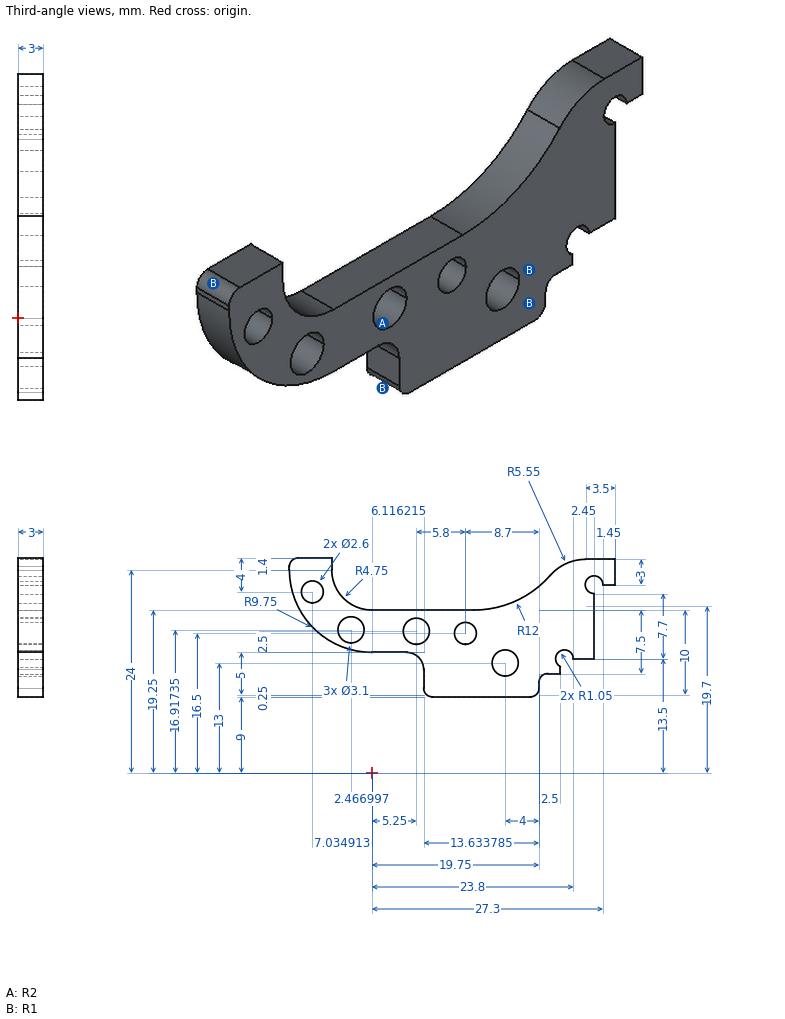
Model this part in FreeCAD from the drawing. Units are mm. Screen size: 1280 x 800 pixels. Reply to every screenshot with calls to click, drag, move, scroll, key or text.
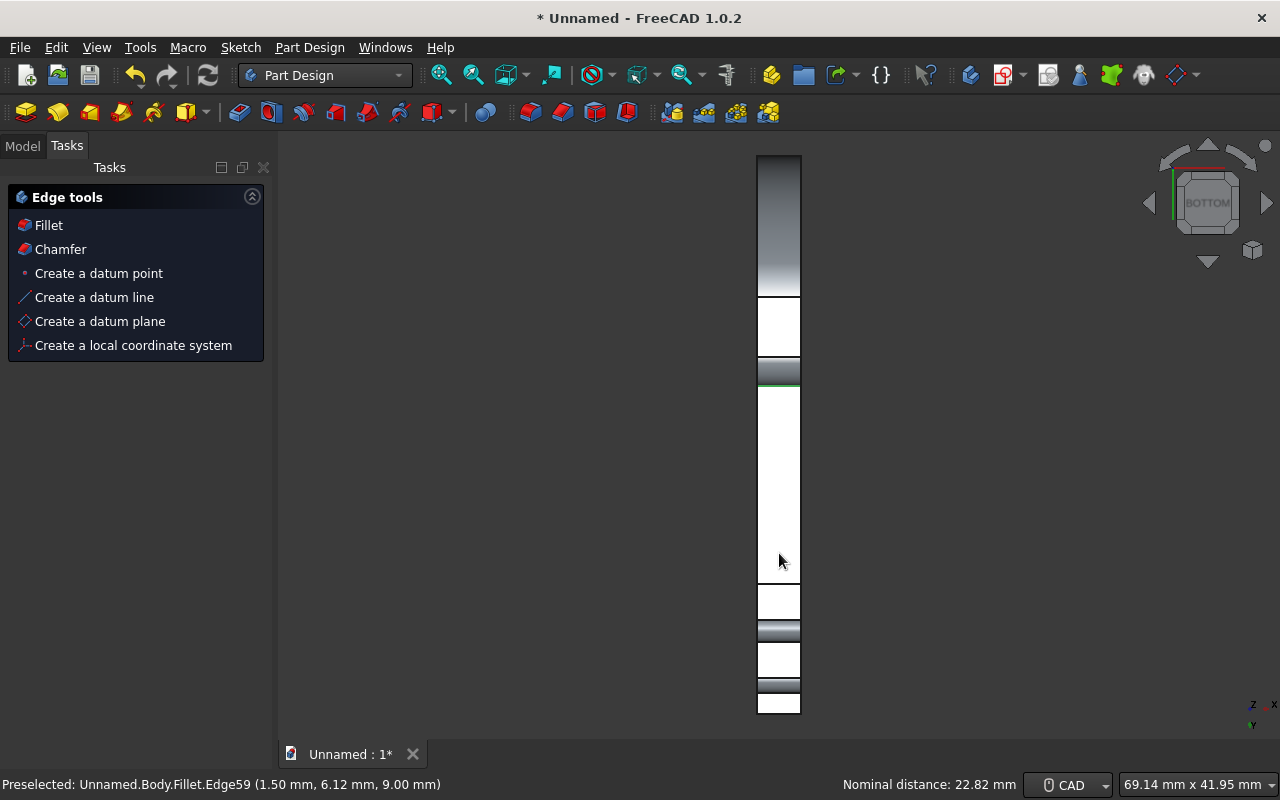
click(779, 583, ctrl)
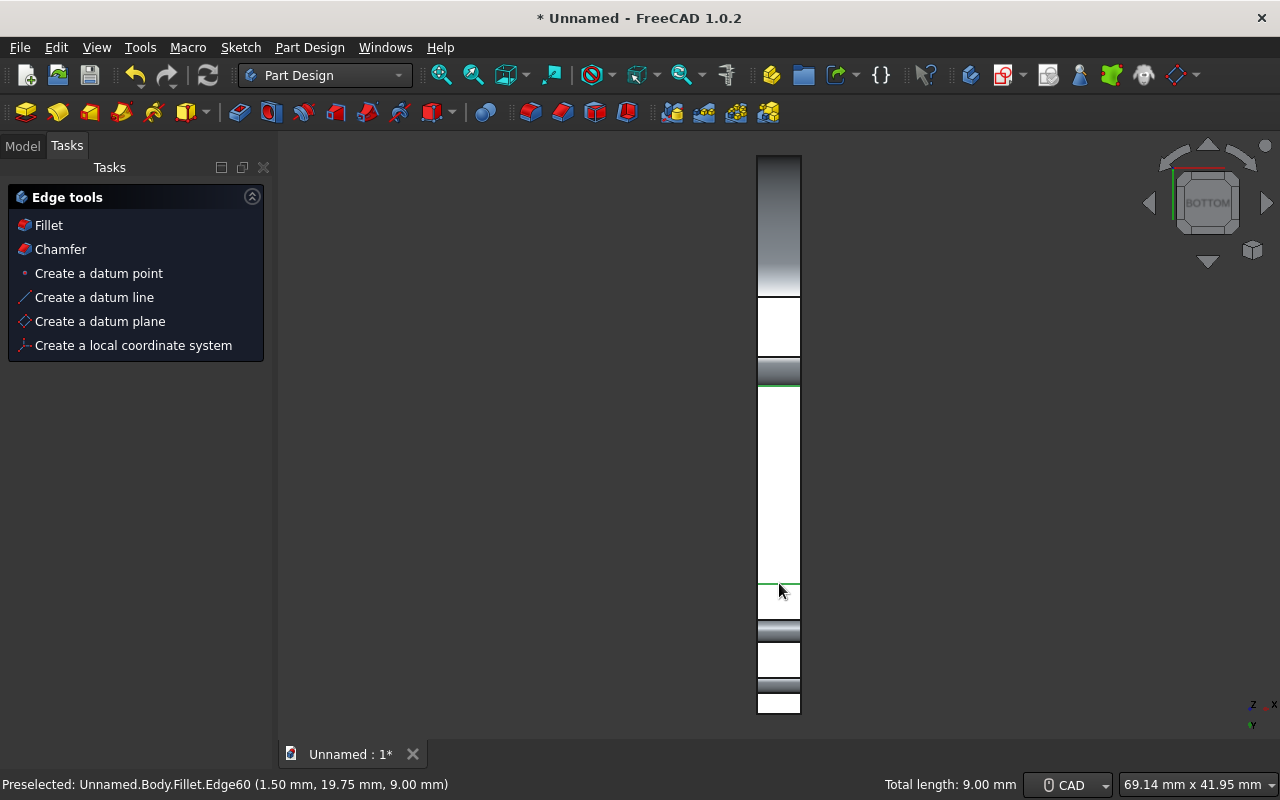
key(4)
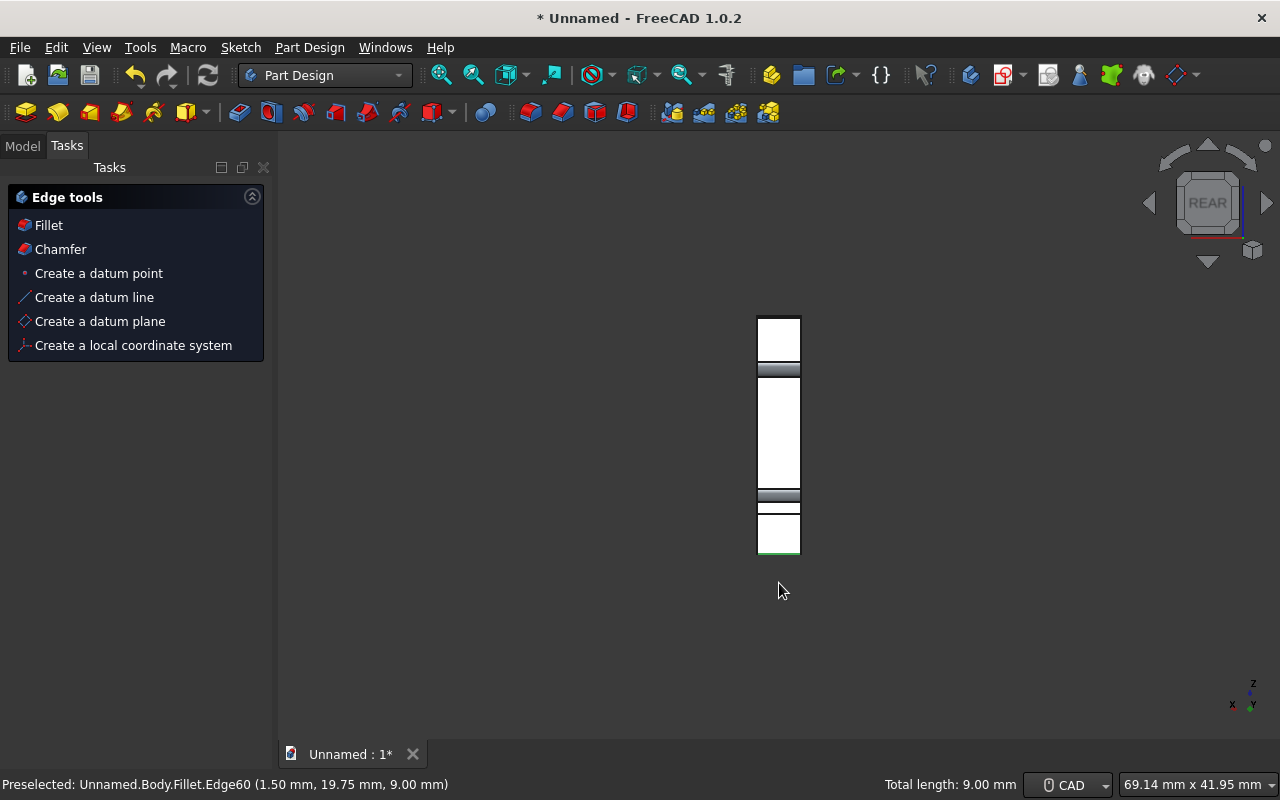
key(v)
key(f)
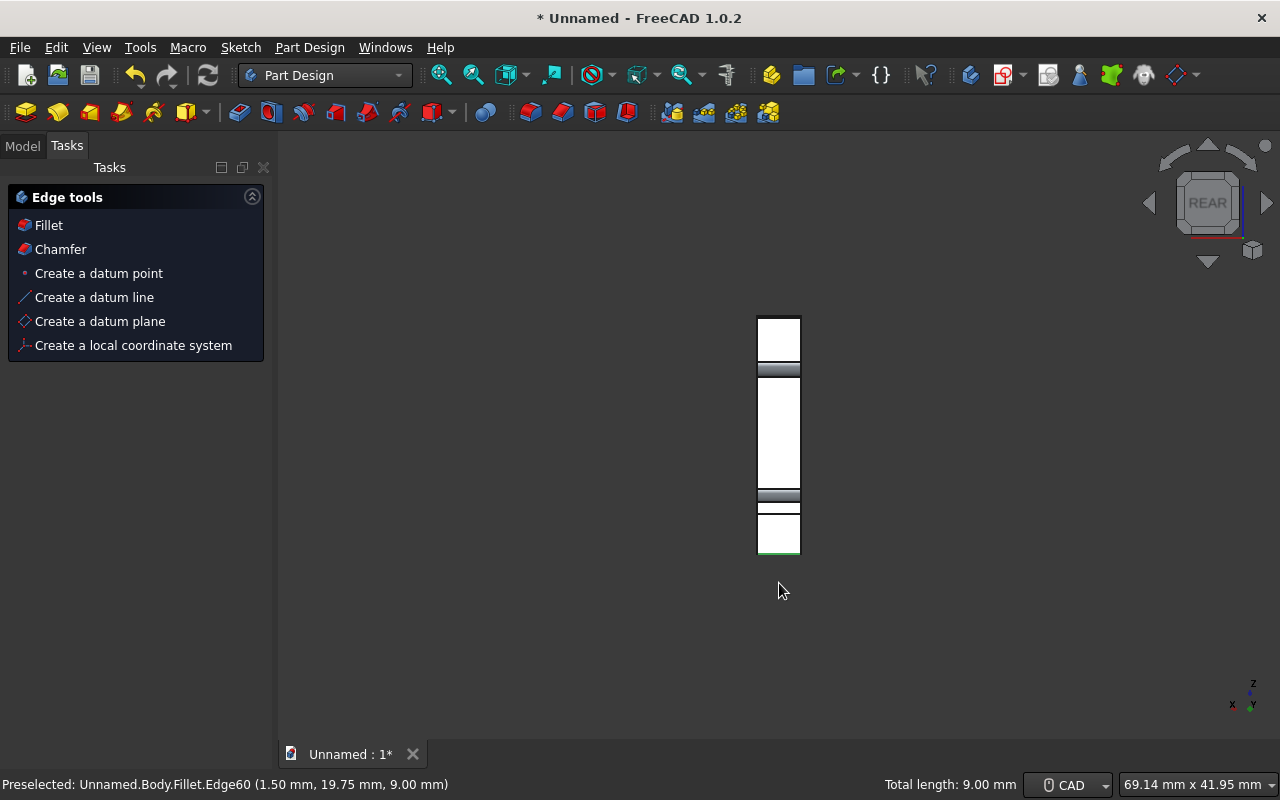
key(6)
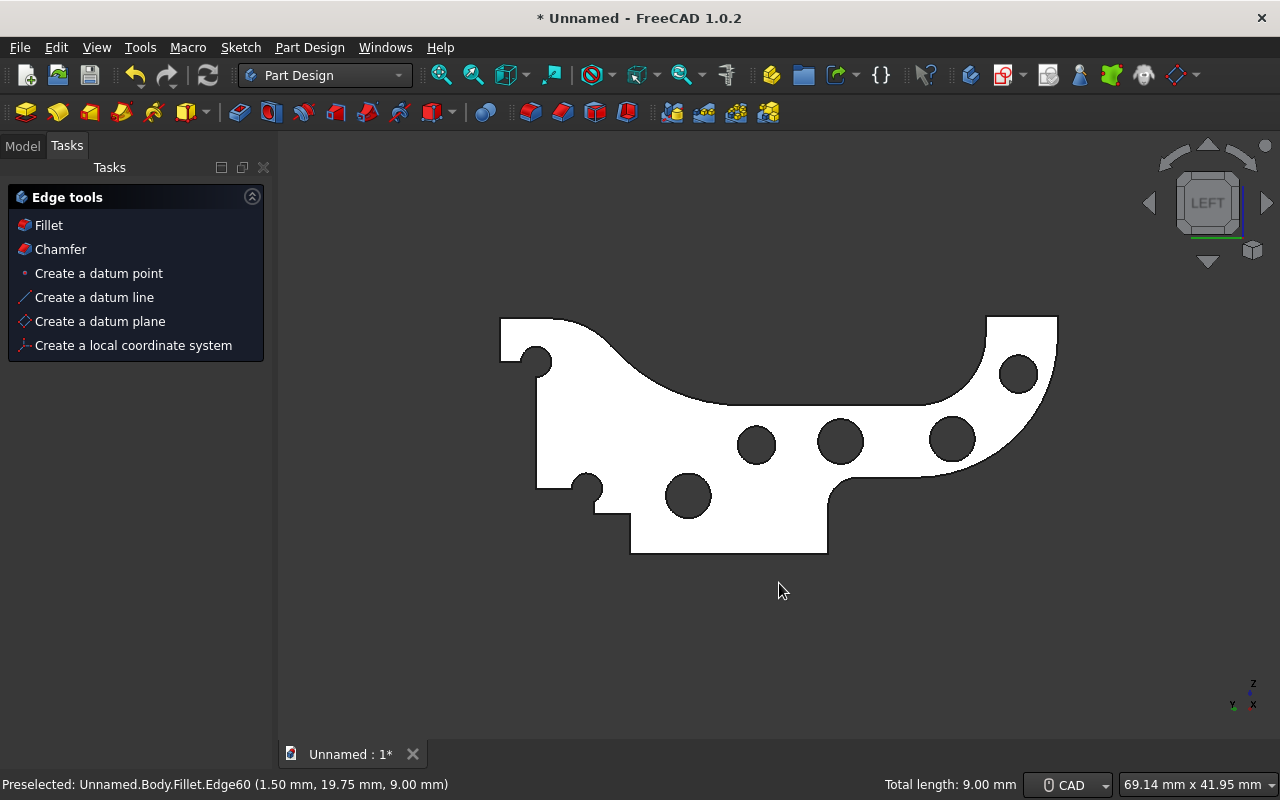
key(v)
key(3)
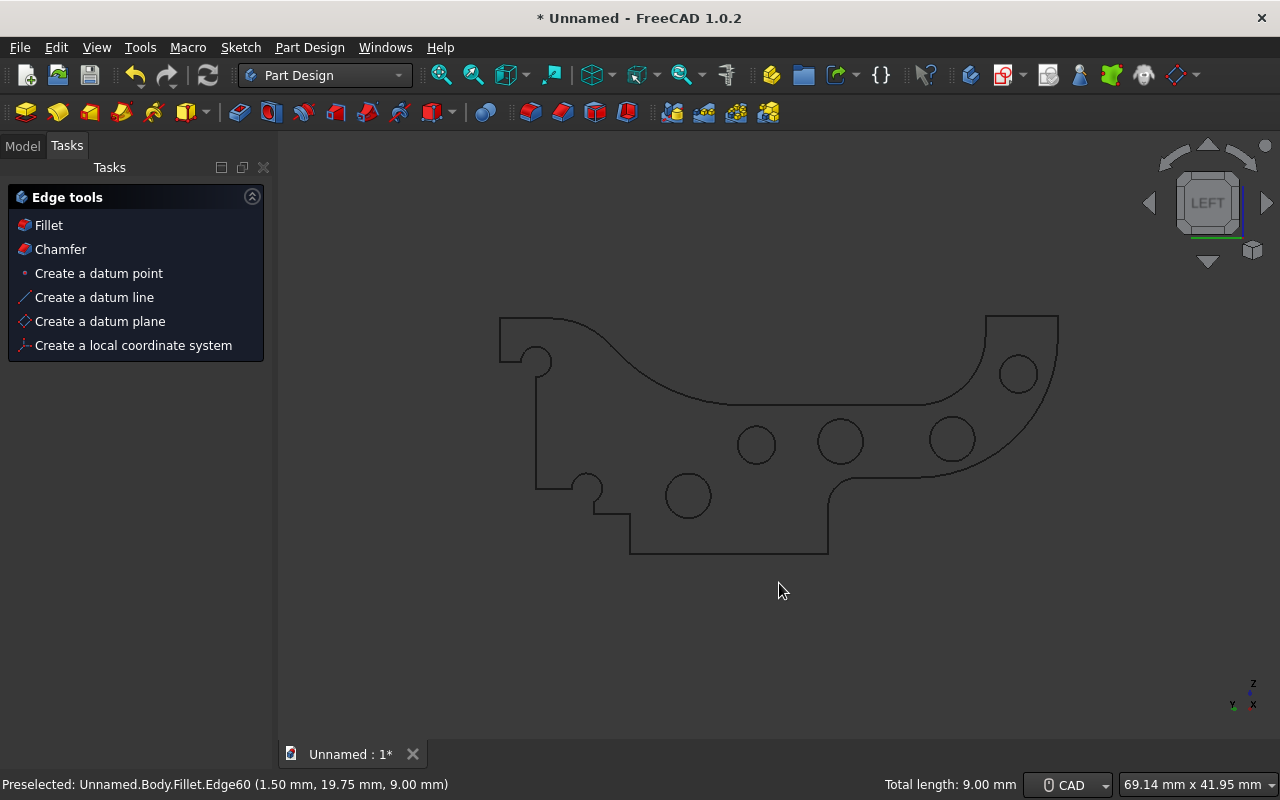
key(0)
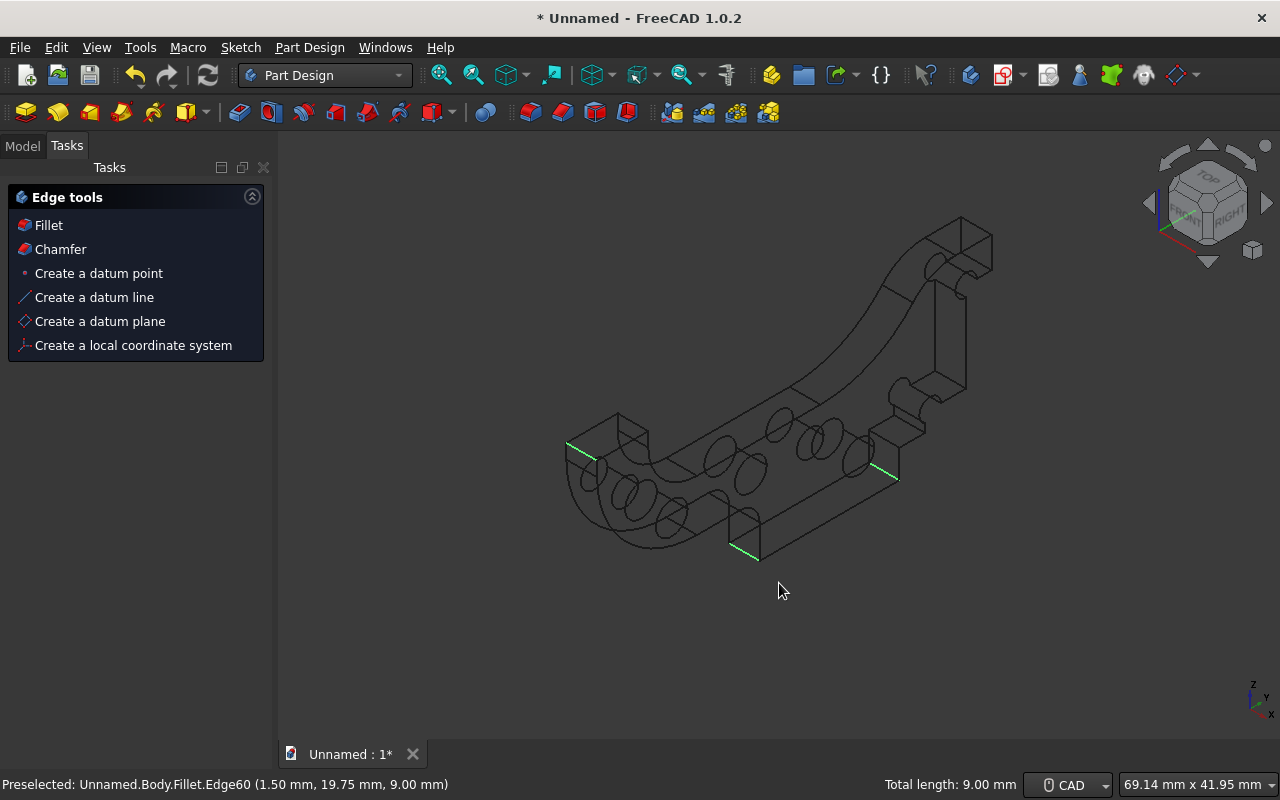
click(884, 438, ctrl)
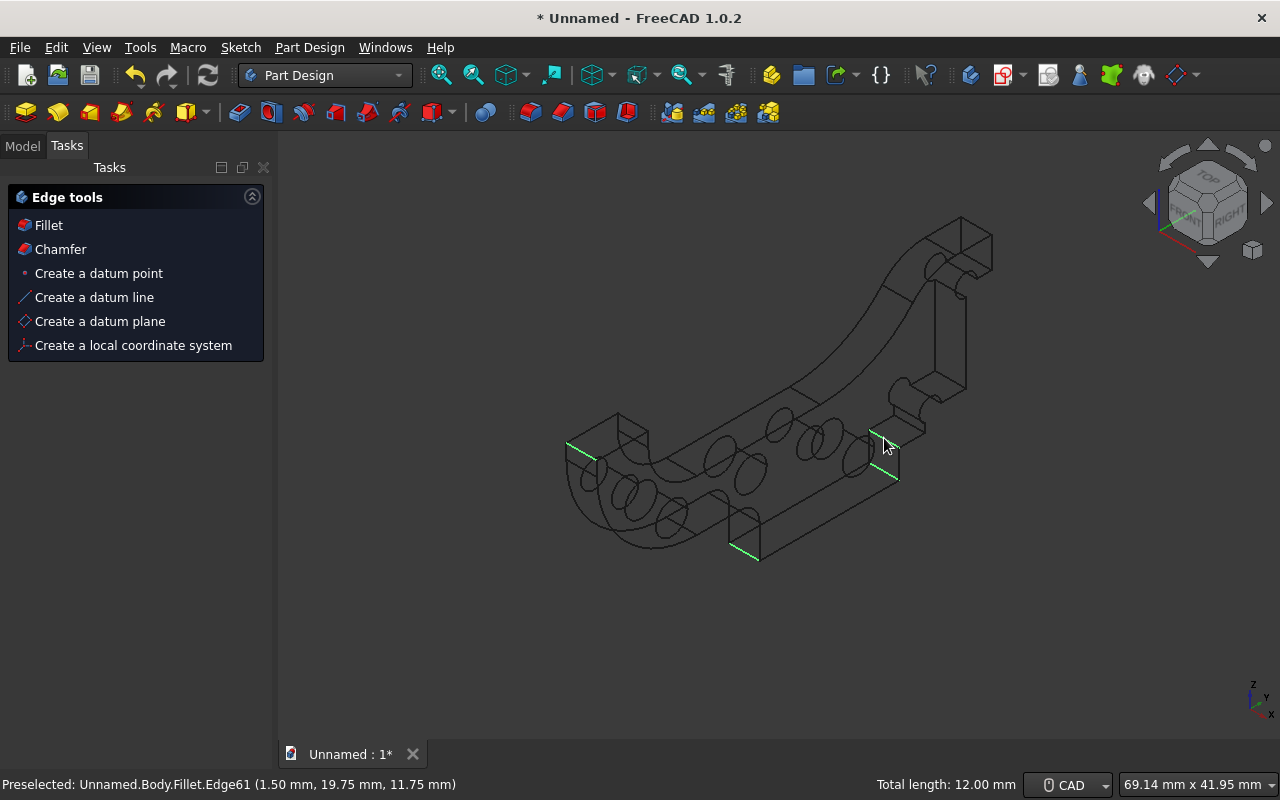
key(v)
key(1)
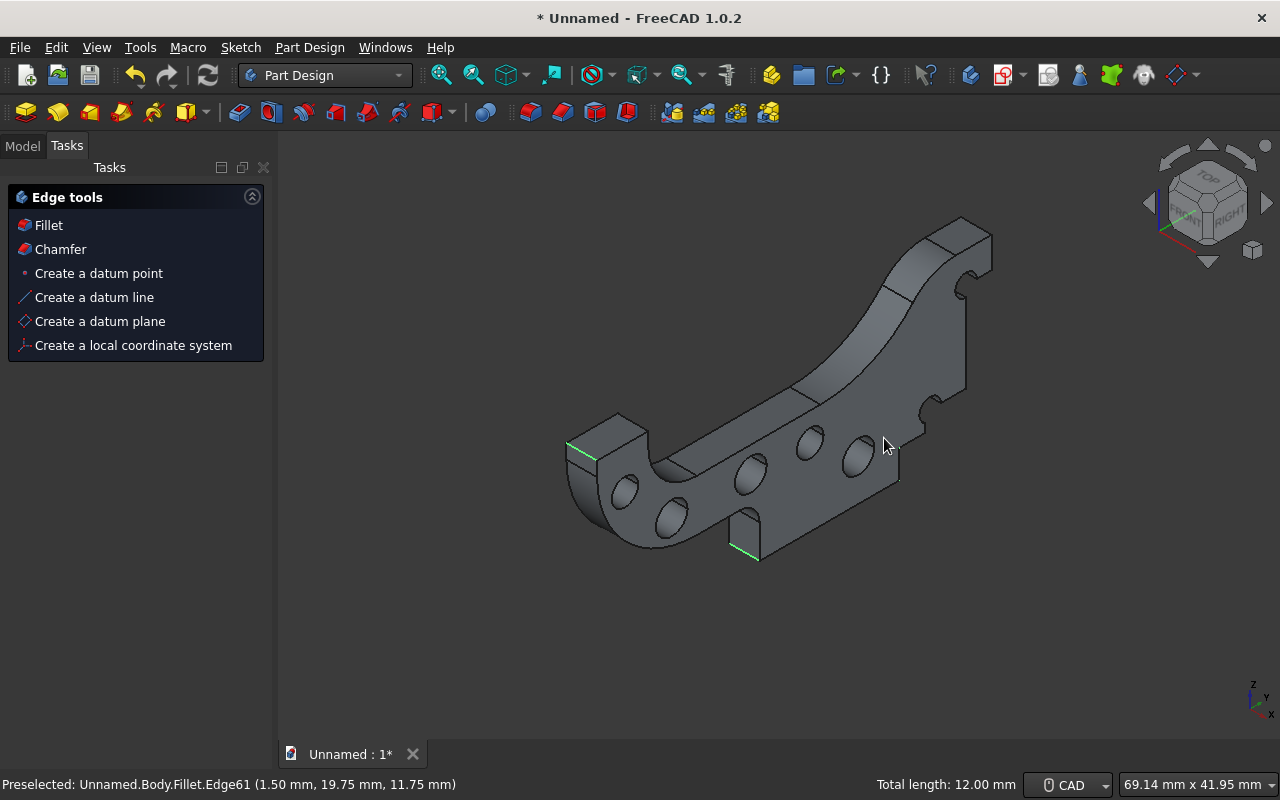
click(532, 112)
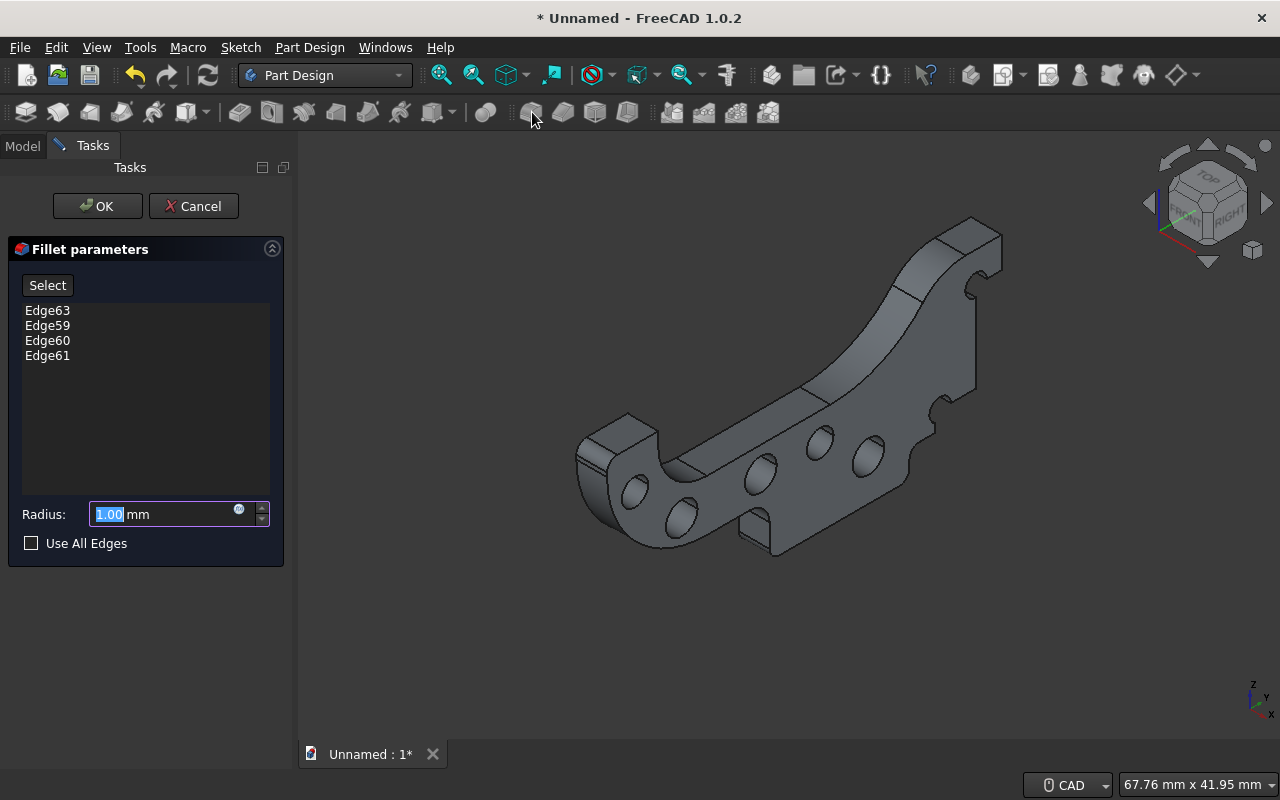
text(1)
key(Tab)